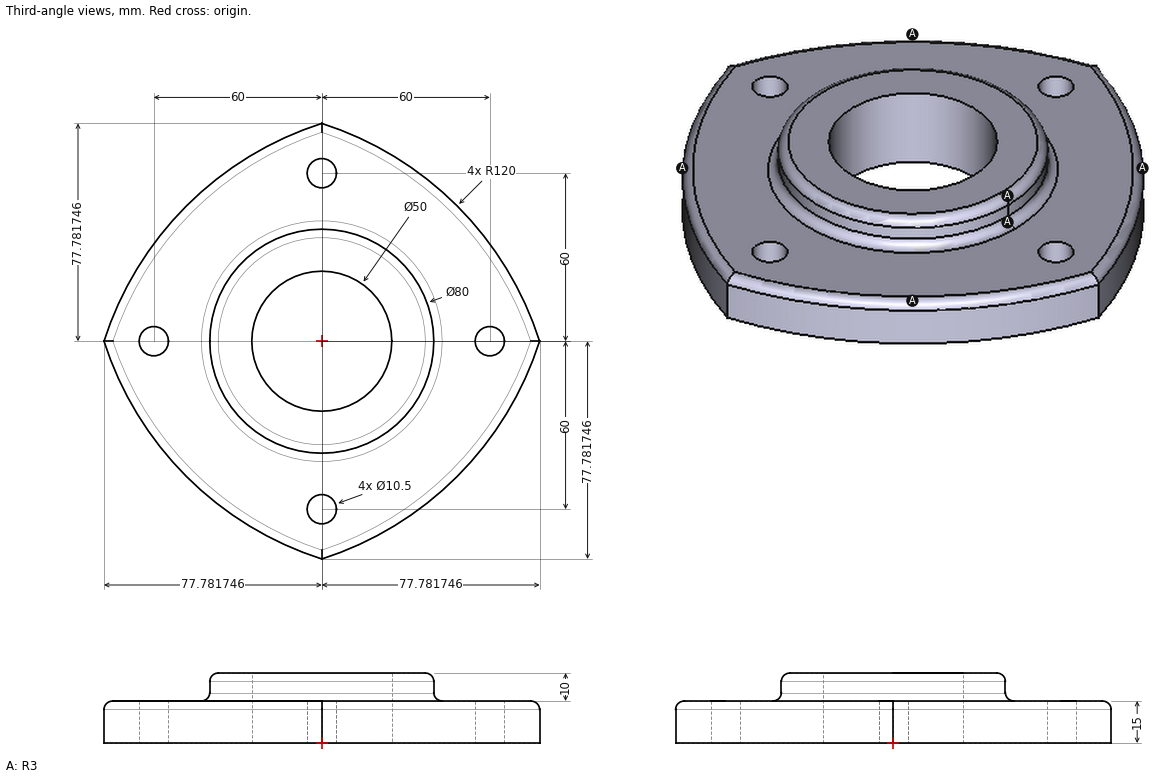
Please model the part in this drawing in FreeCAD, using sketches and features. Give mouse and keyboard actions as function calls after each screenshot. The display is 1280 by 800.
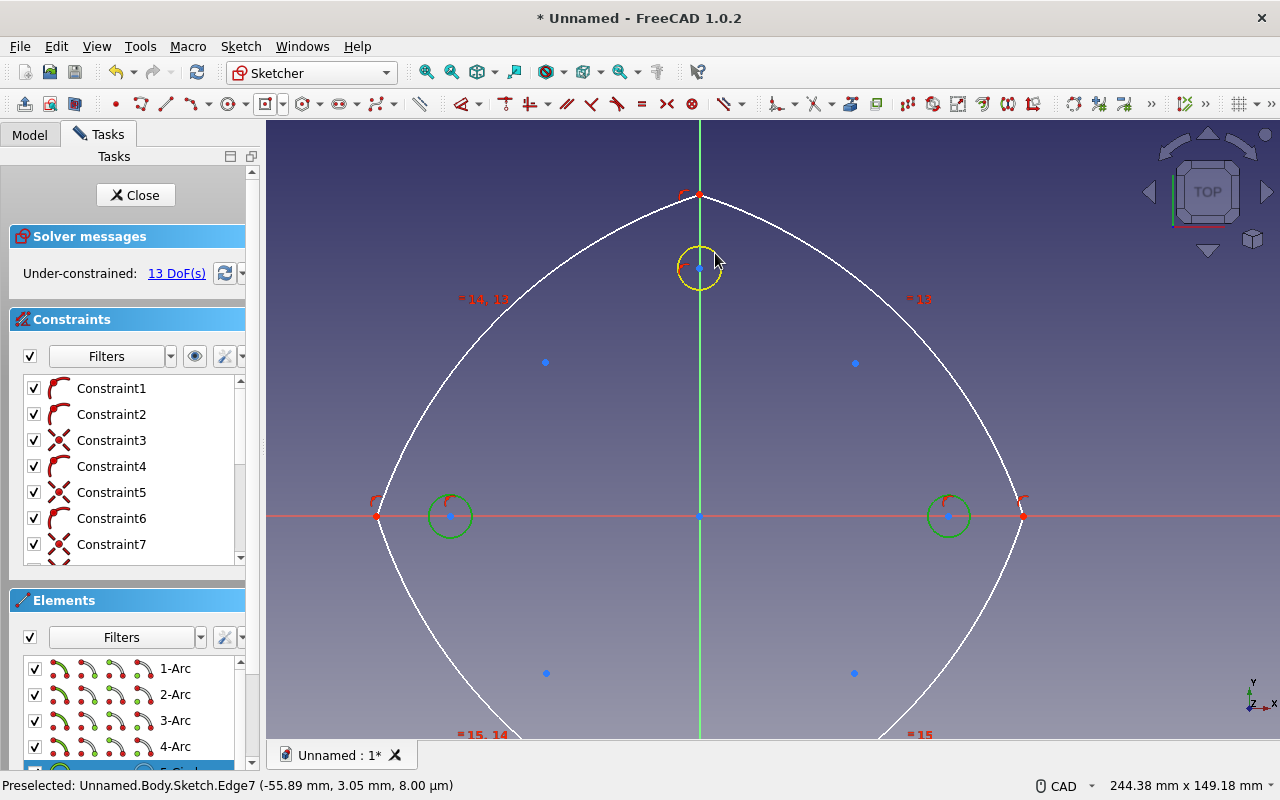
click(715, 253)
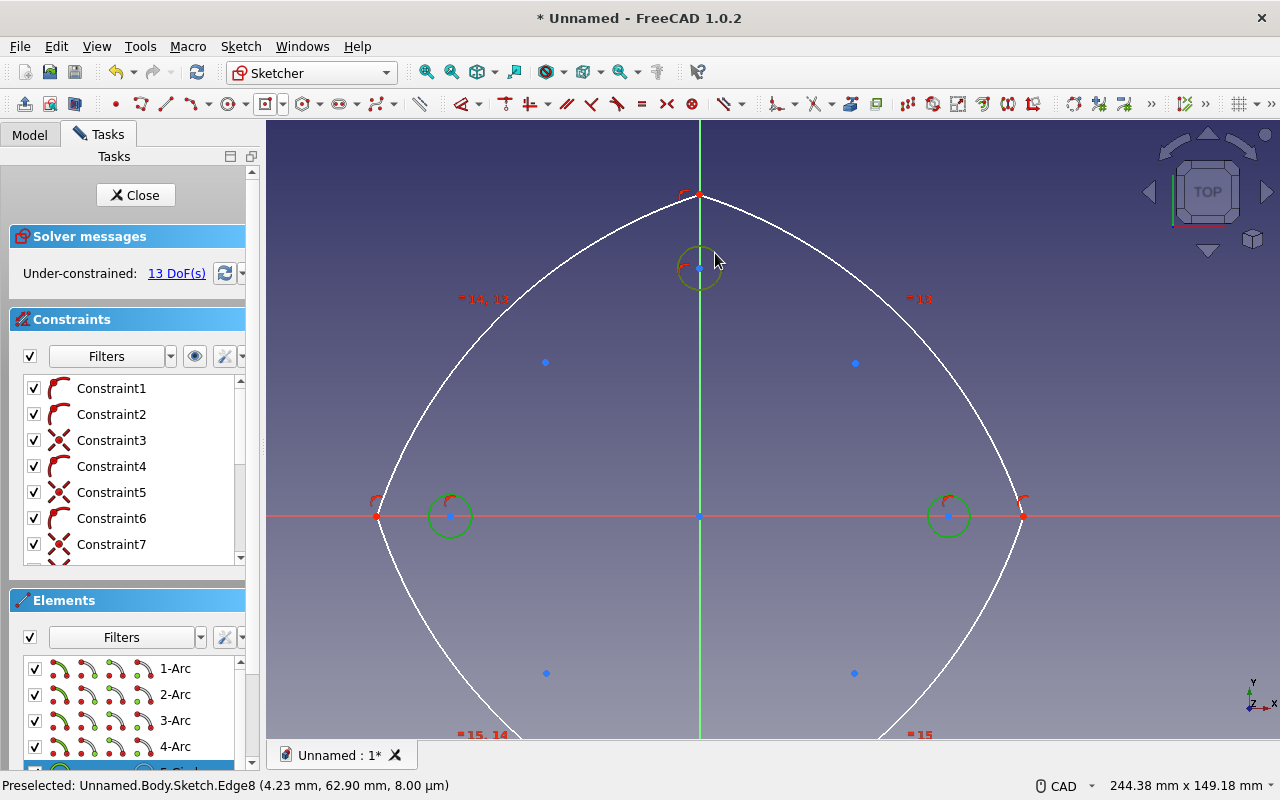
click(642, 104)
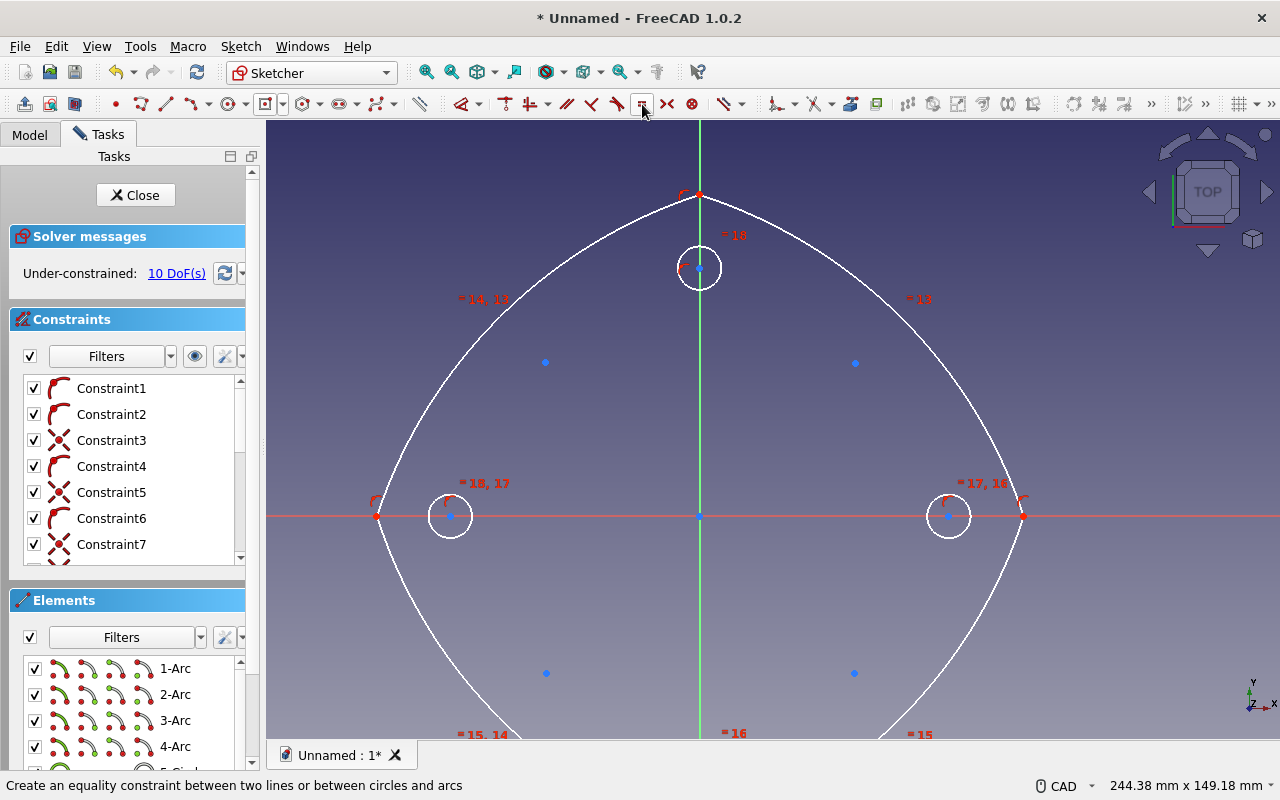
click(460, 104)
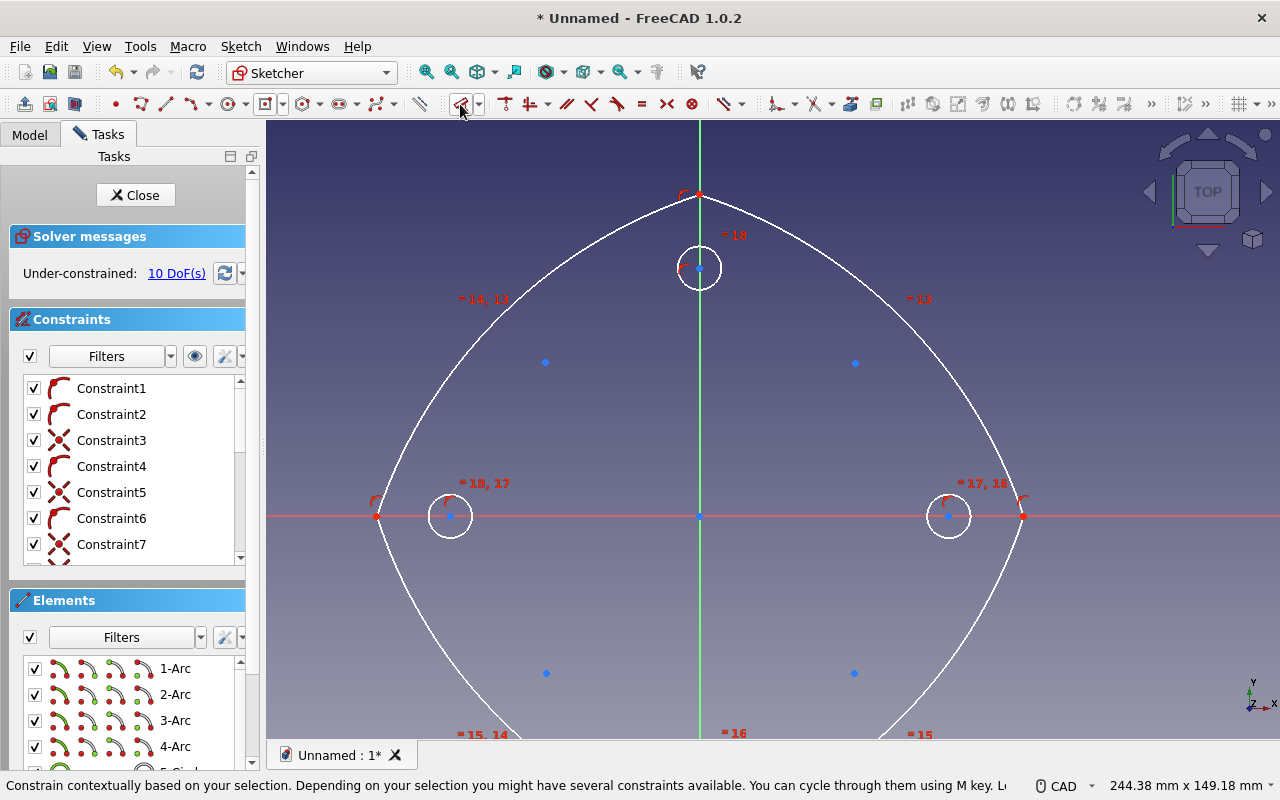
click(961, 389)
click(987, 371)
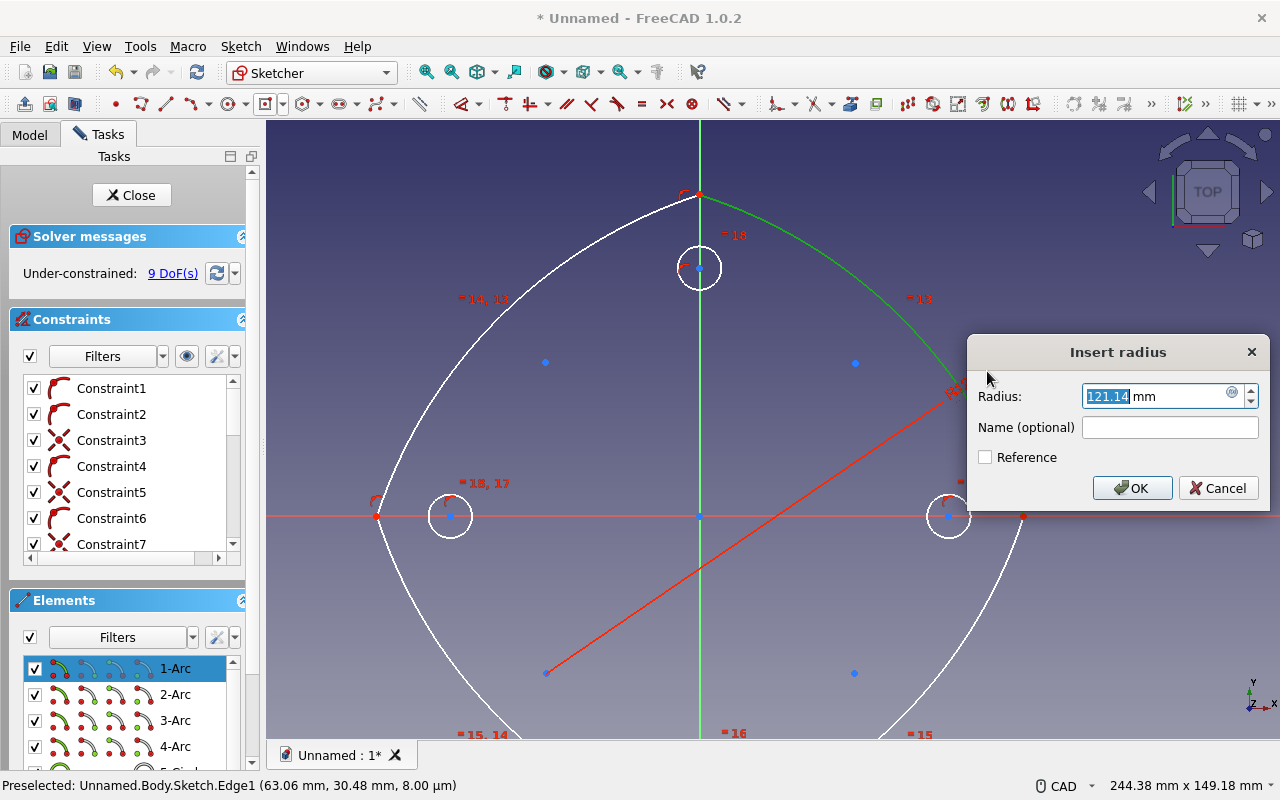
text(120)
key(Return)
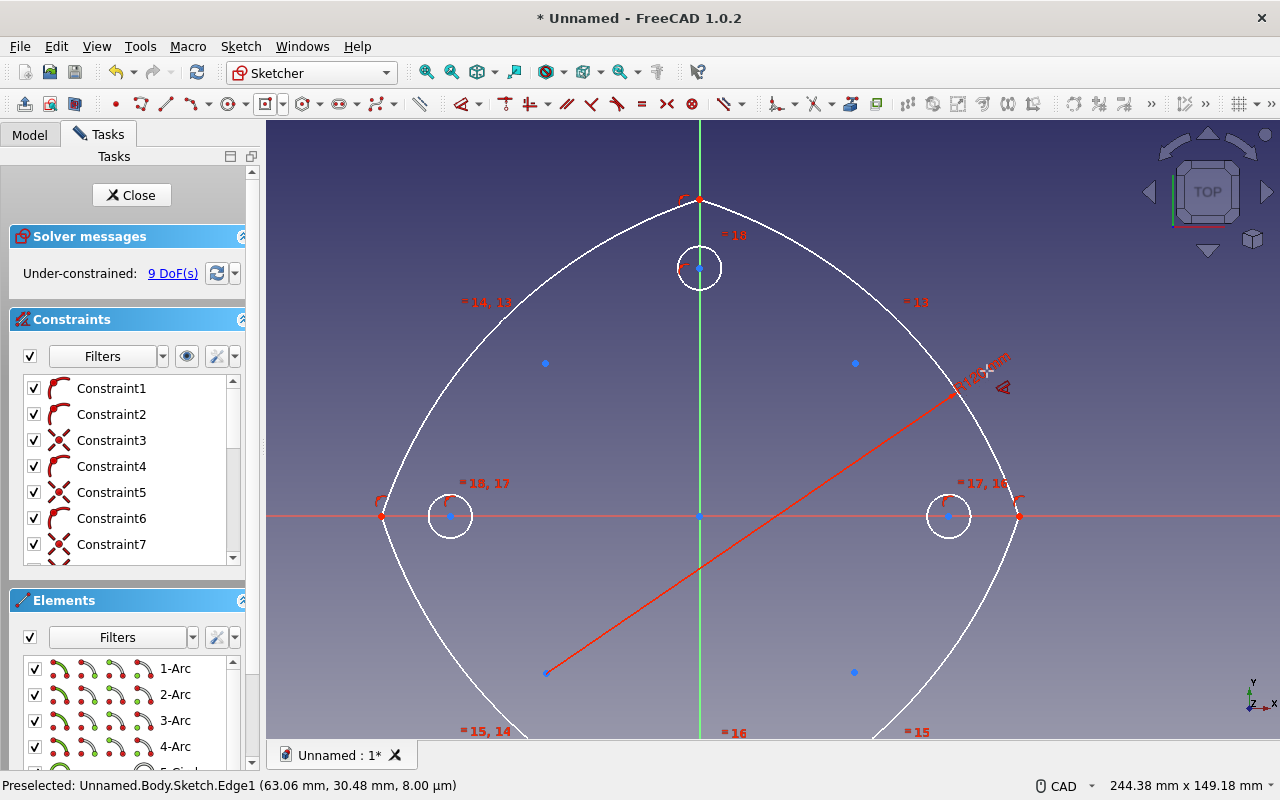
scroll(715, 253, down, 2)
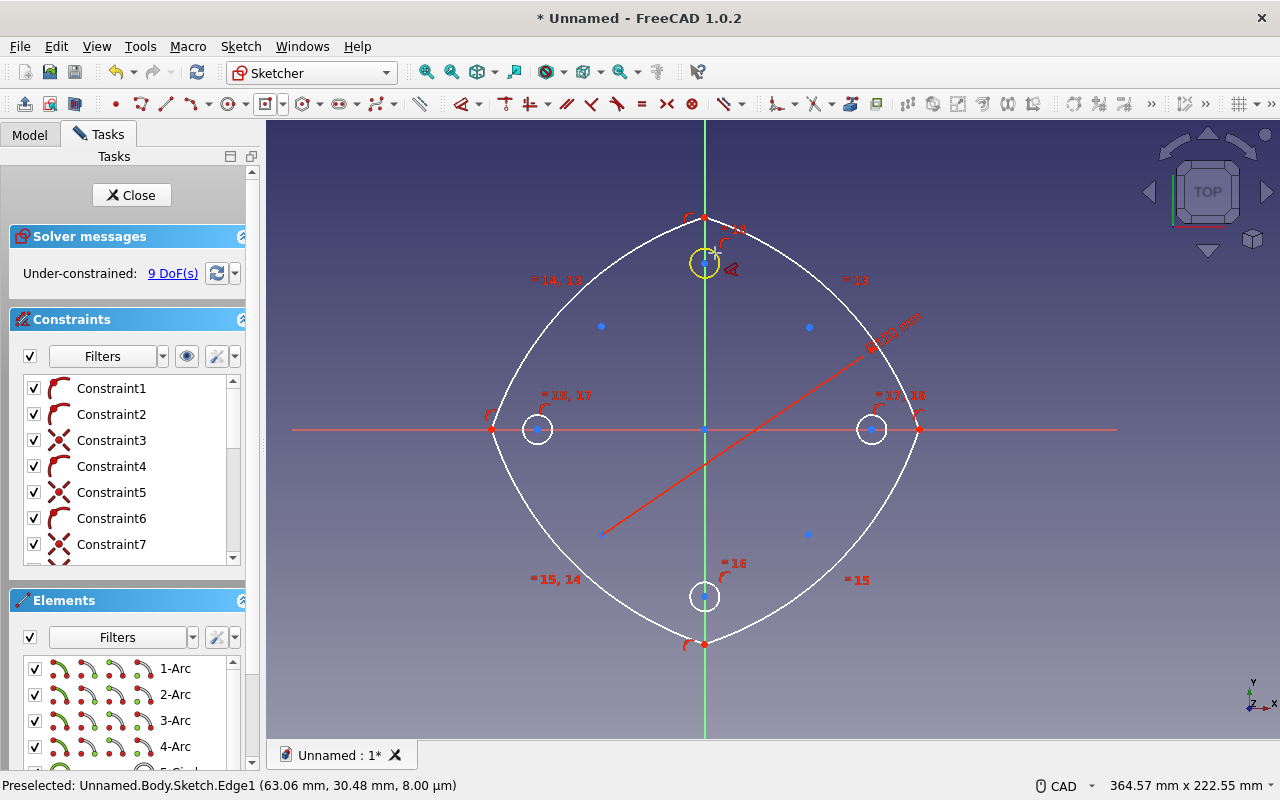
scroll(715, 587, up, 2)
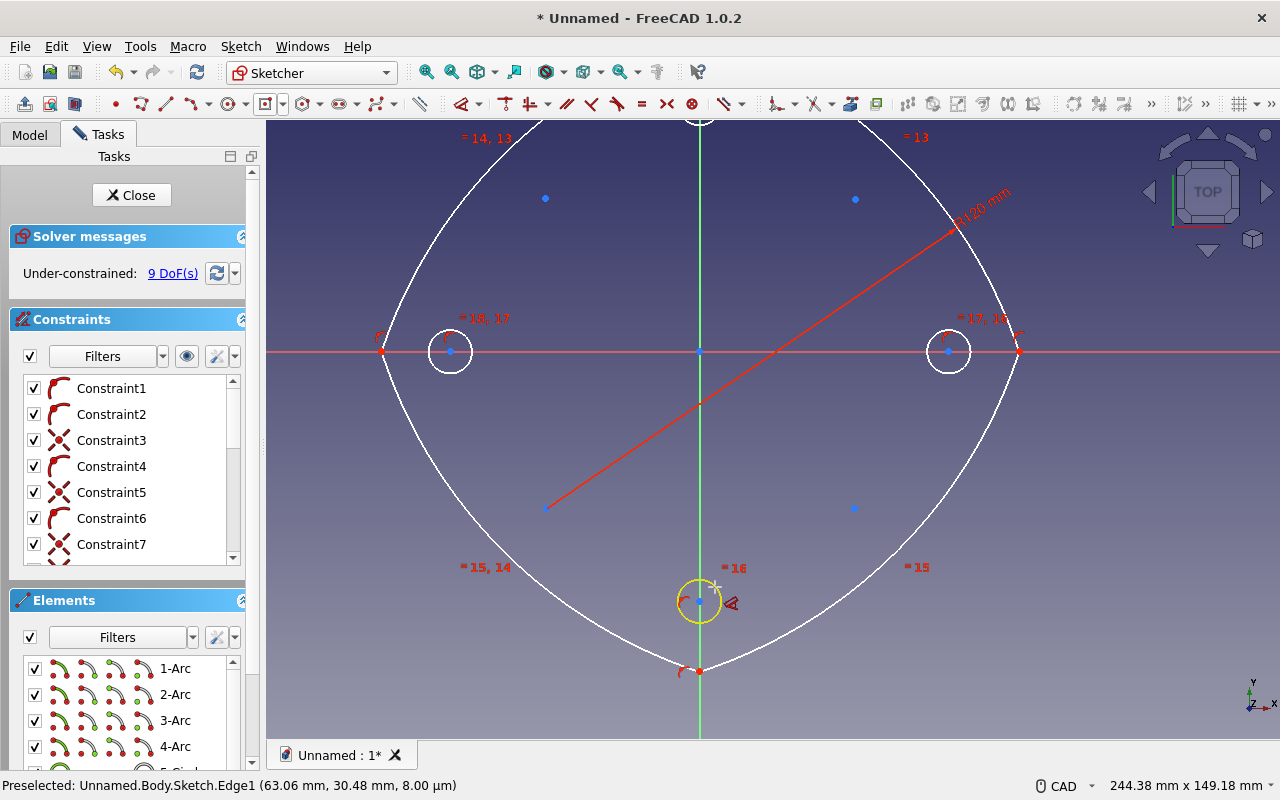
click(715, 586)
click(738, 563)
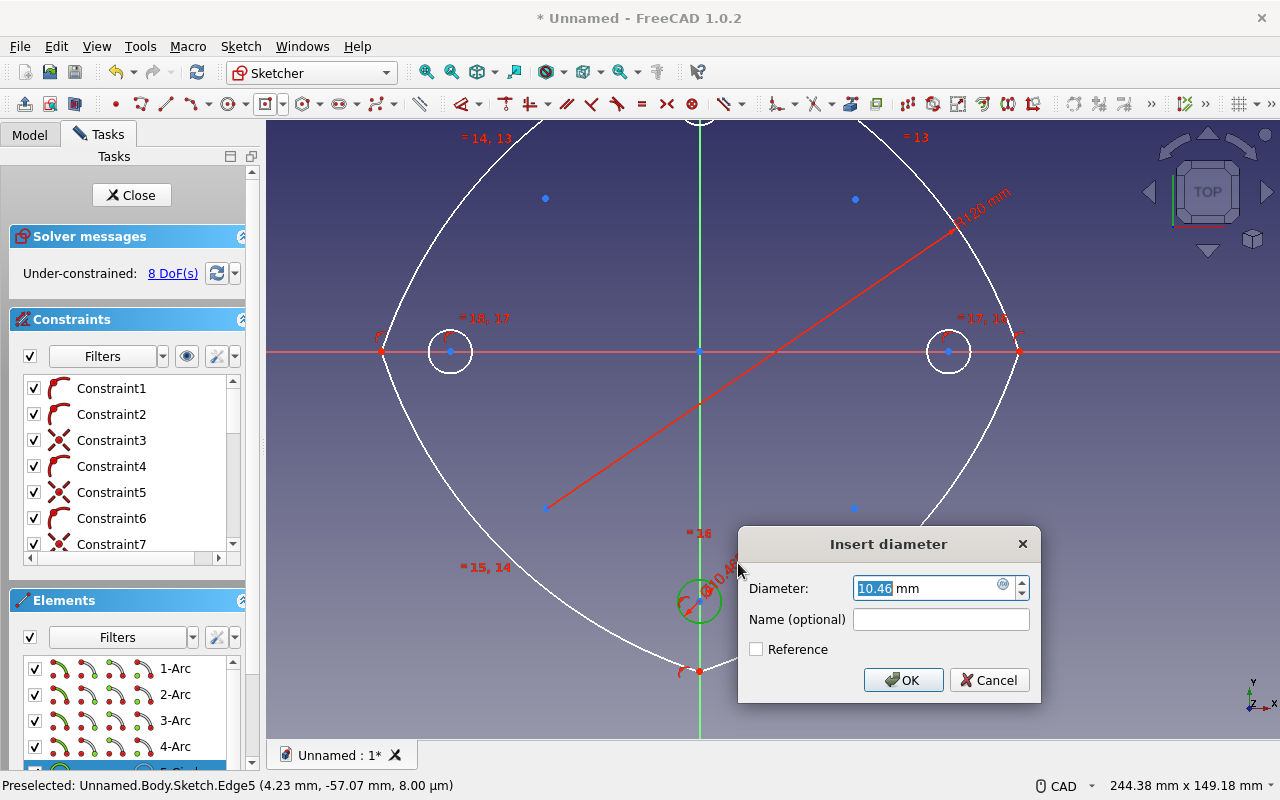
text(10.5)
key(Return)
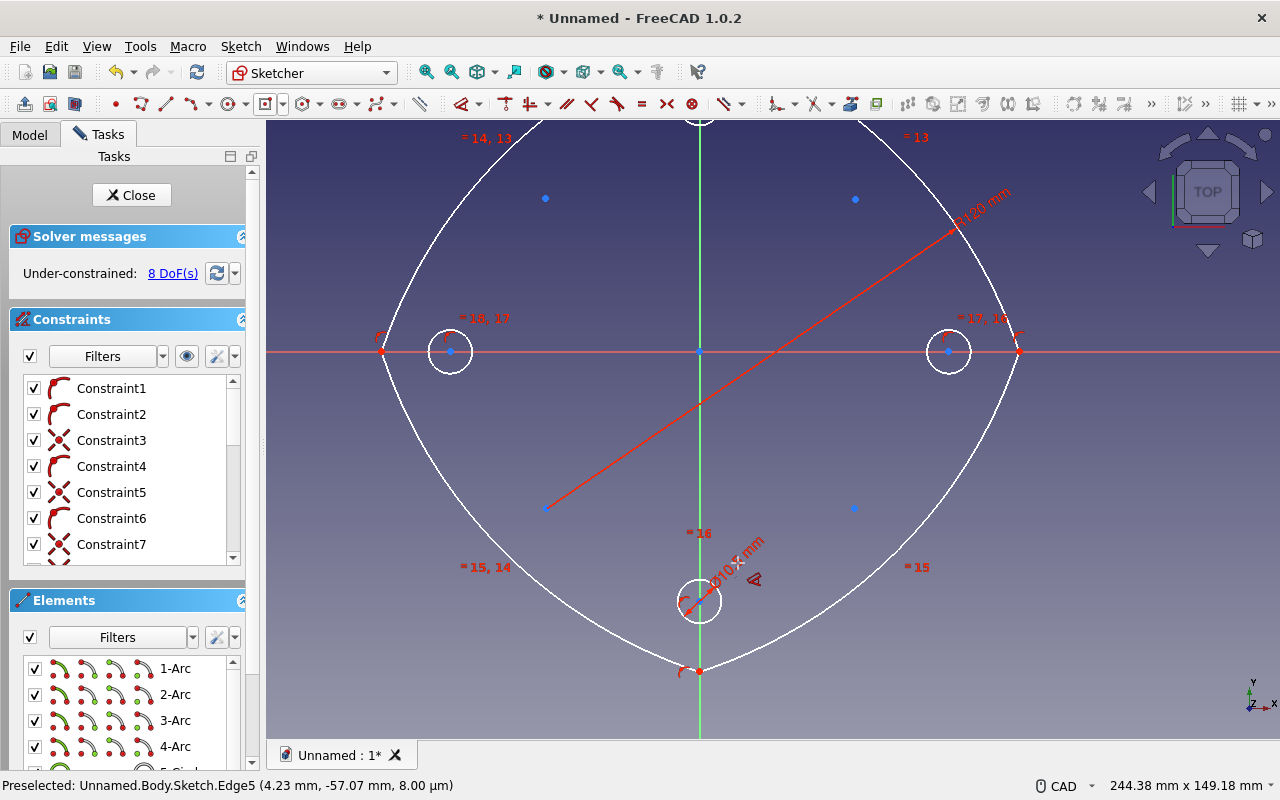
click(700, 601)
click(734, 477)